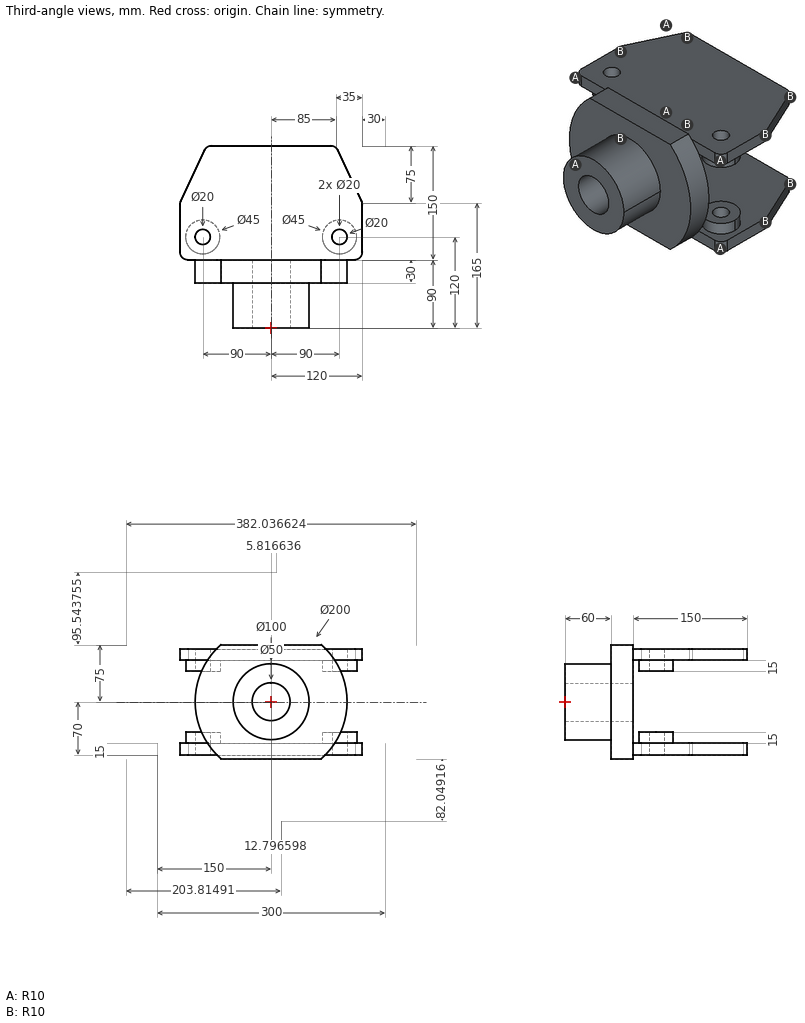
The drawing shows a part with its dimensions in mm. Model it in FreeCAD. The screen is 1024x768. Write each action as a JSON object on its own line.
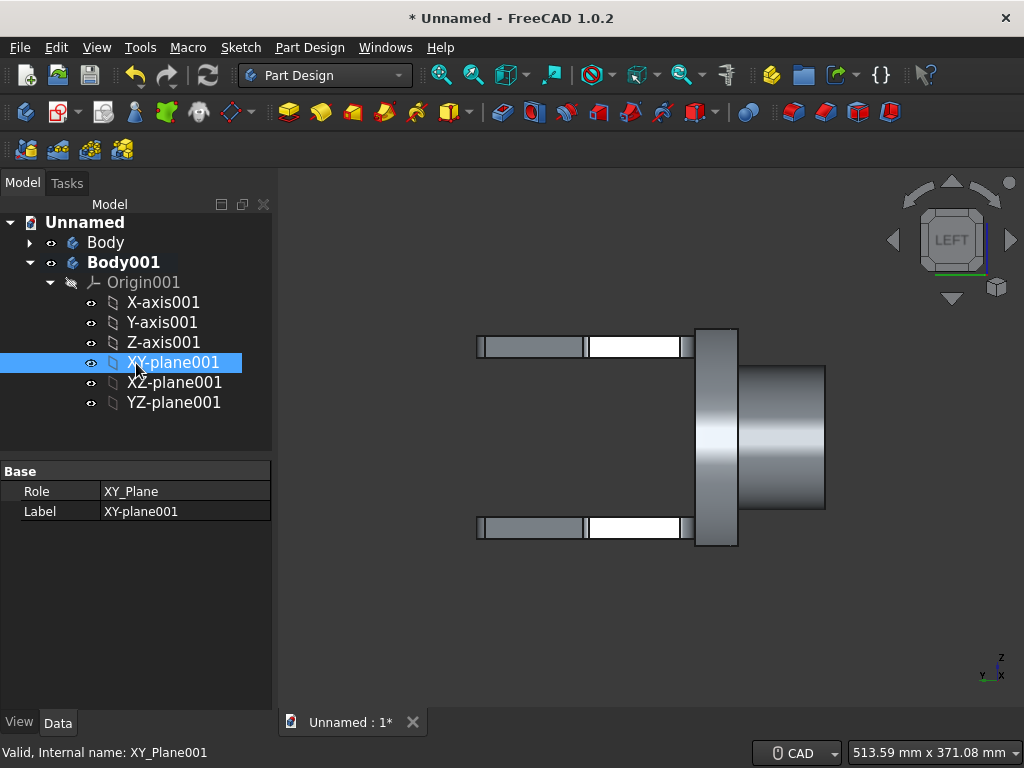
{"action": "left_click", "coordinate": [232, 112]}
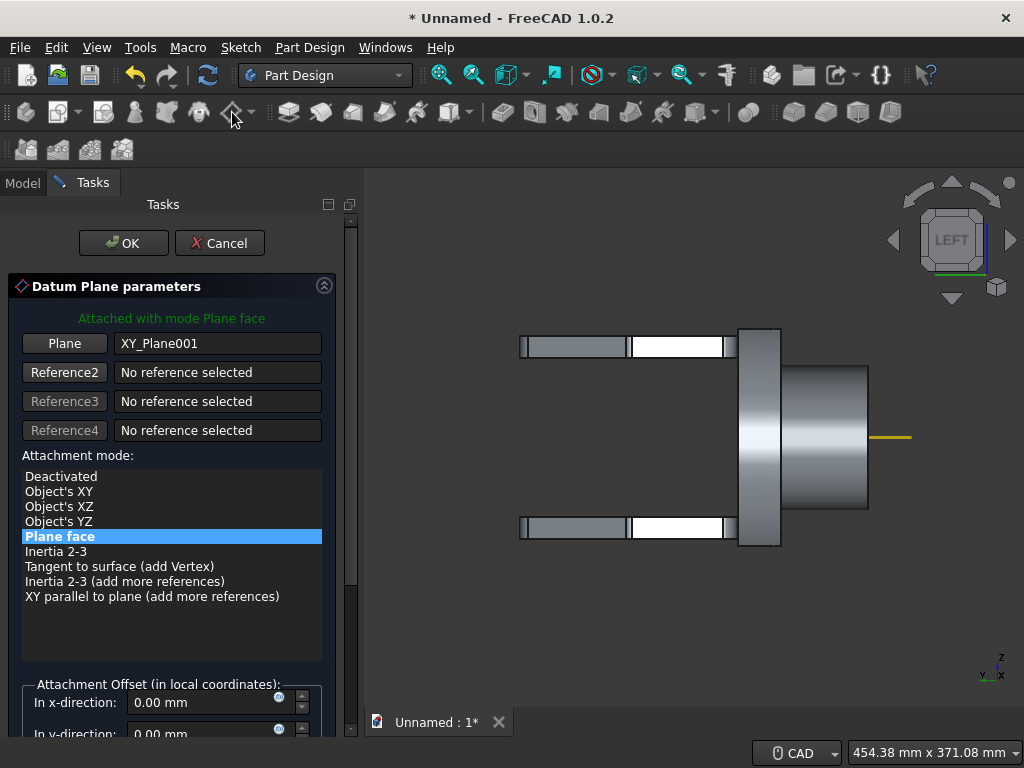
{"action": "scroll", "coordinate": [351, 475], "scroll_direction": "down", "scroll_amount": 2}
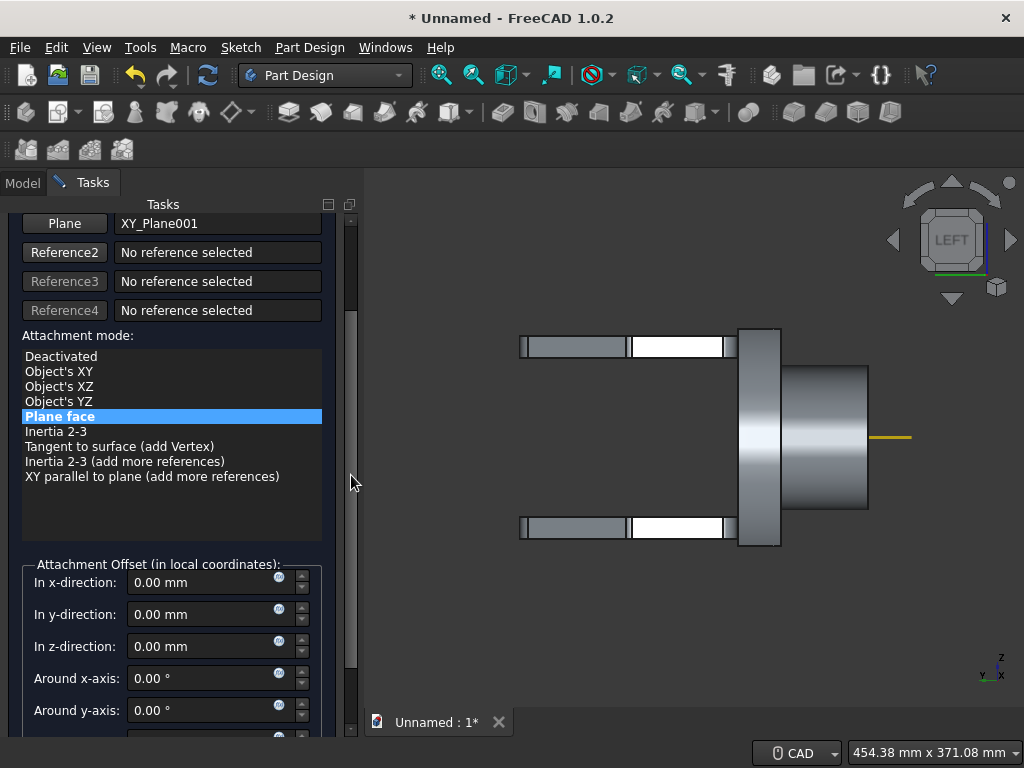
{"action": "triple_click", "coordinate": [210, 646]}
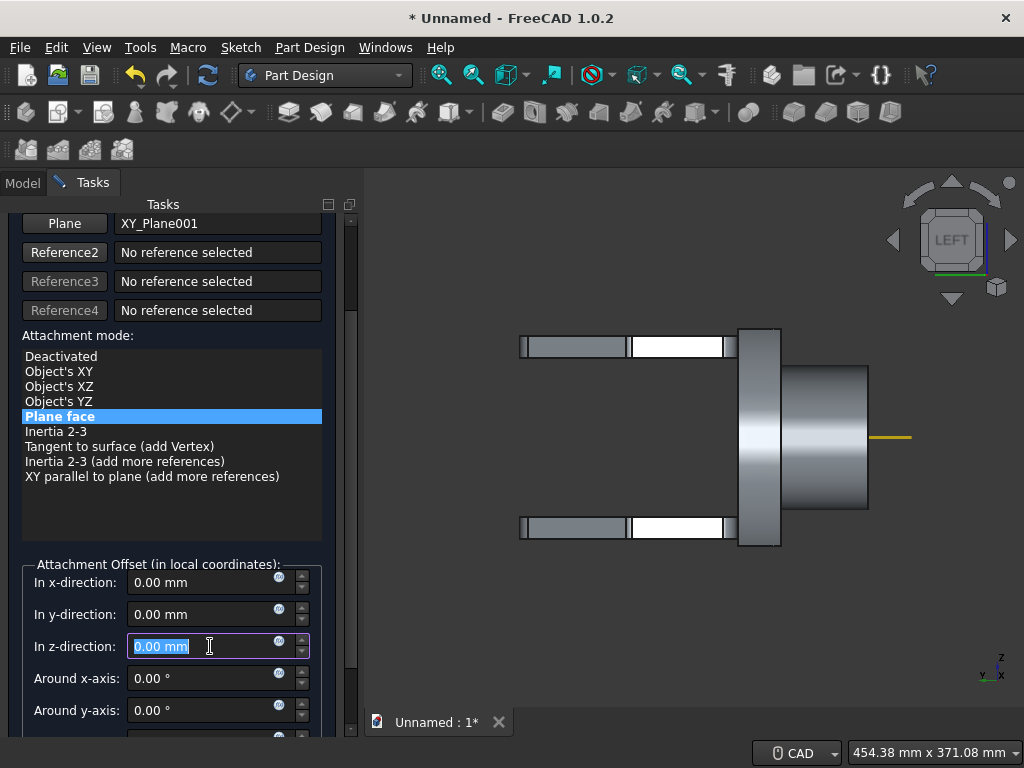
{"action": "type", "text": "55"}
{"action": "key", "text": "Tab"}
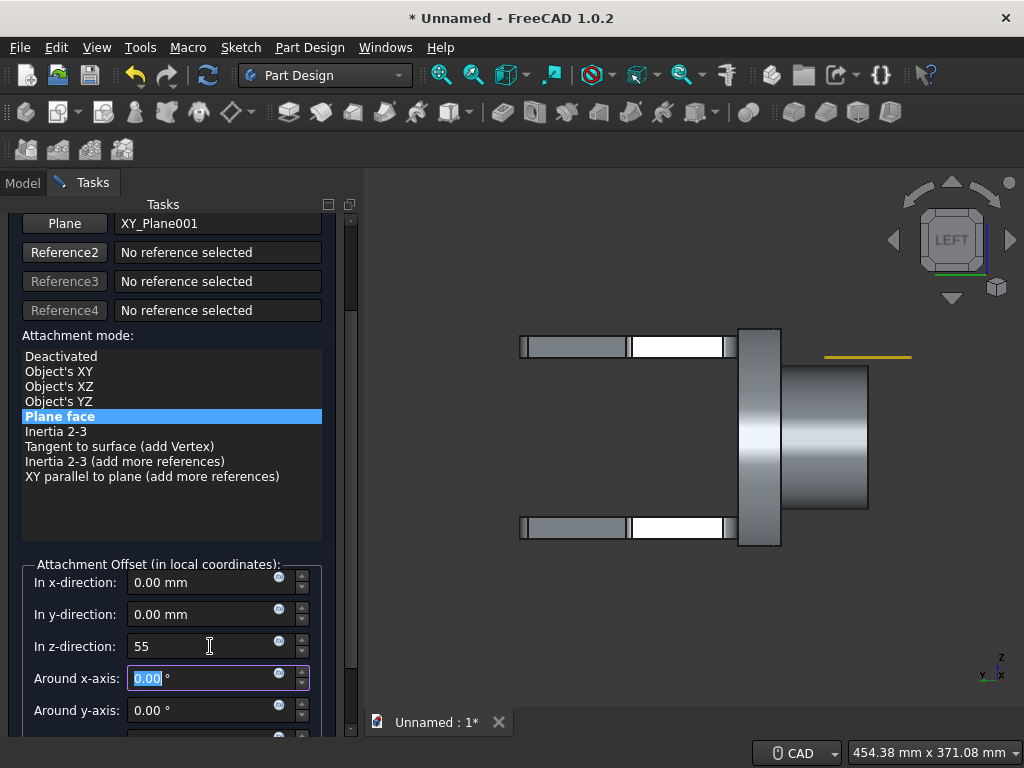
{"action": "scroll", "coordinate": [351, 475], "scroll_direction": "up", "scroll_amount": 3}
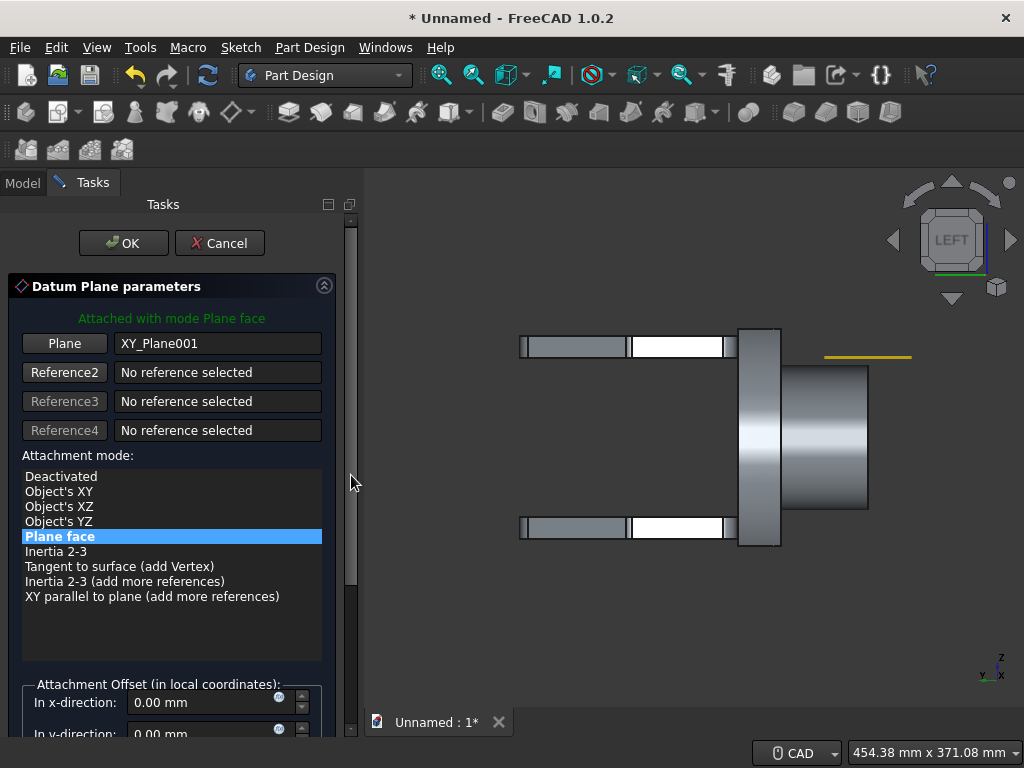
{"action": "left_click", "coordinate": [124, 243]}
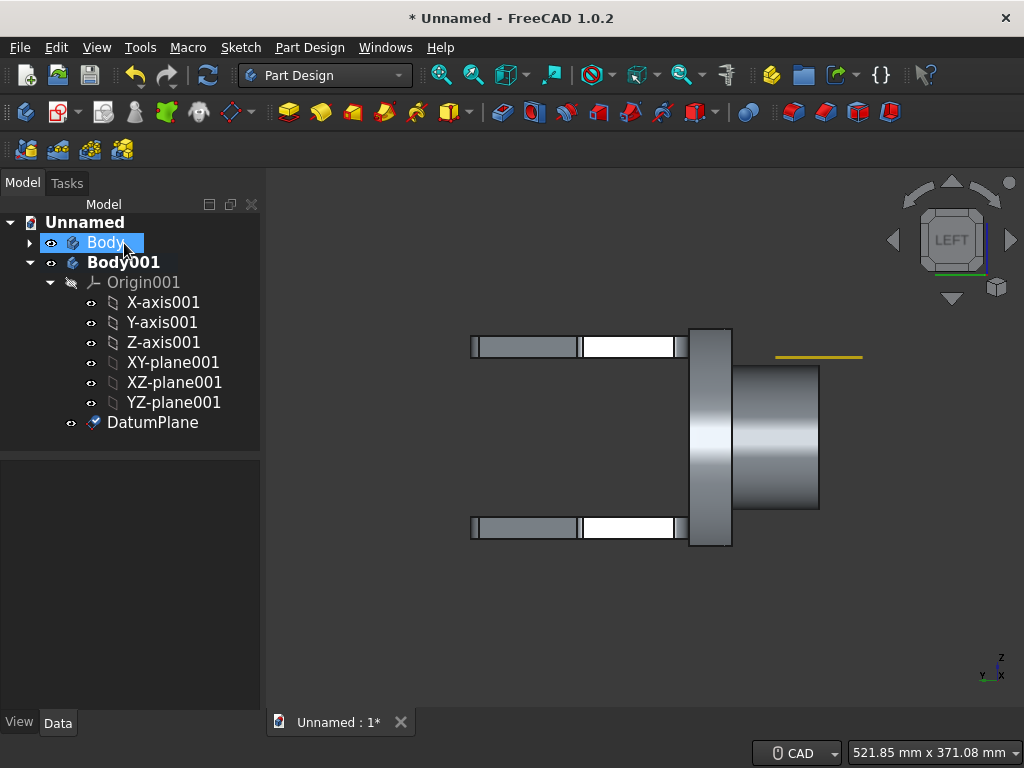
{"action": "left_click", "coordinate": [116, 423]}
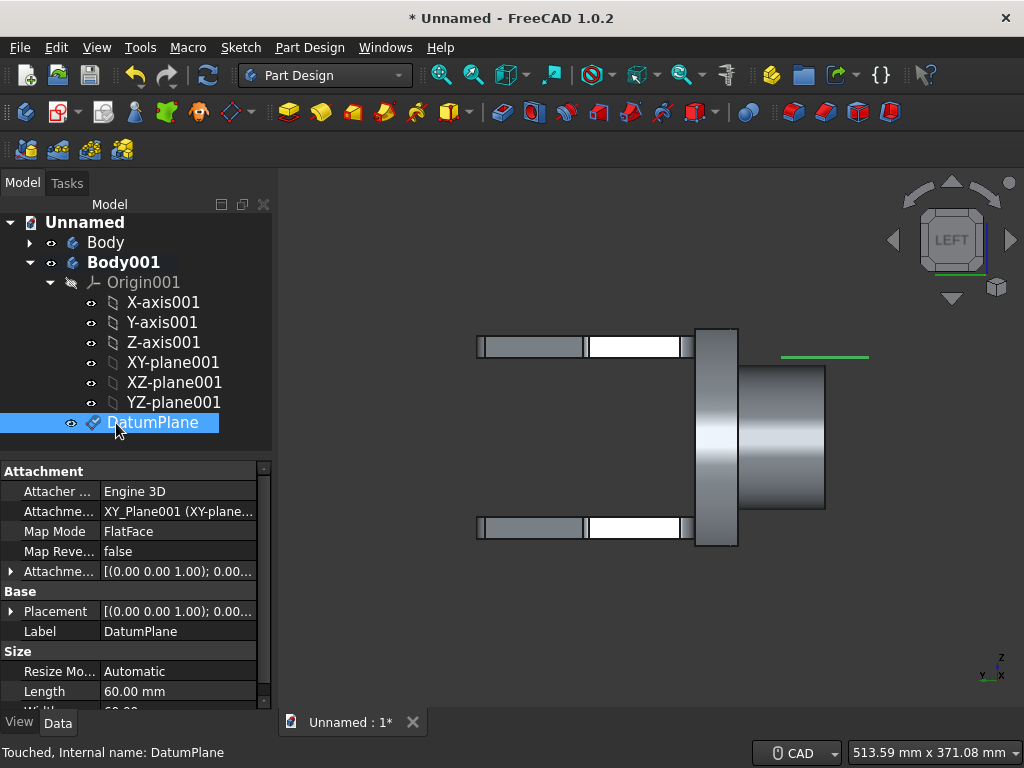
{"action": "left_click", "coordinate": [58, 112]}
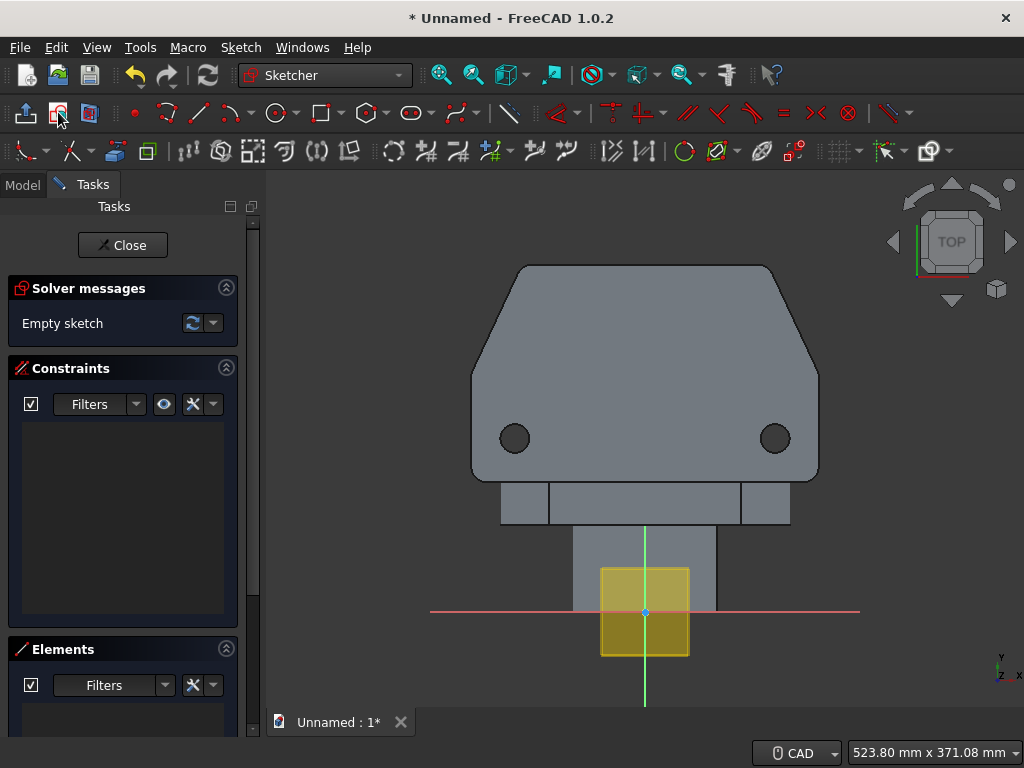
{"action": "scroll", "coordinate": [499, 439], "scroll_direction": "up", "scroll_amount": 8}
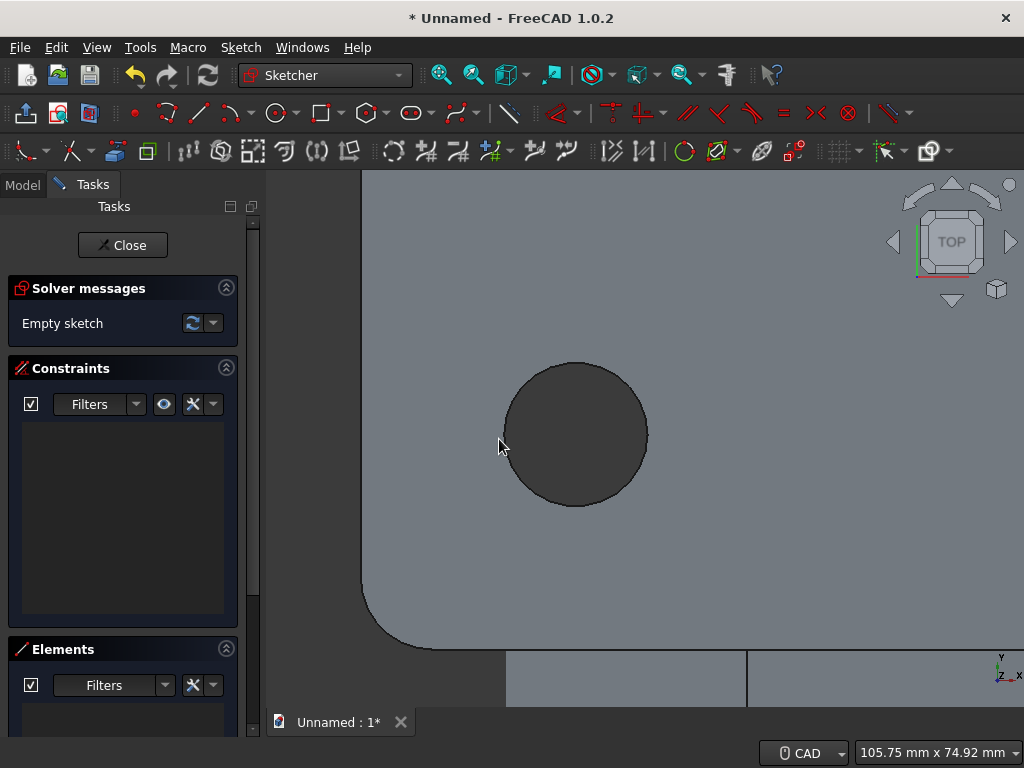
{"action": "key", "text": "g c"}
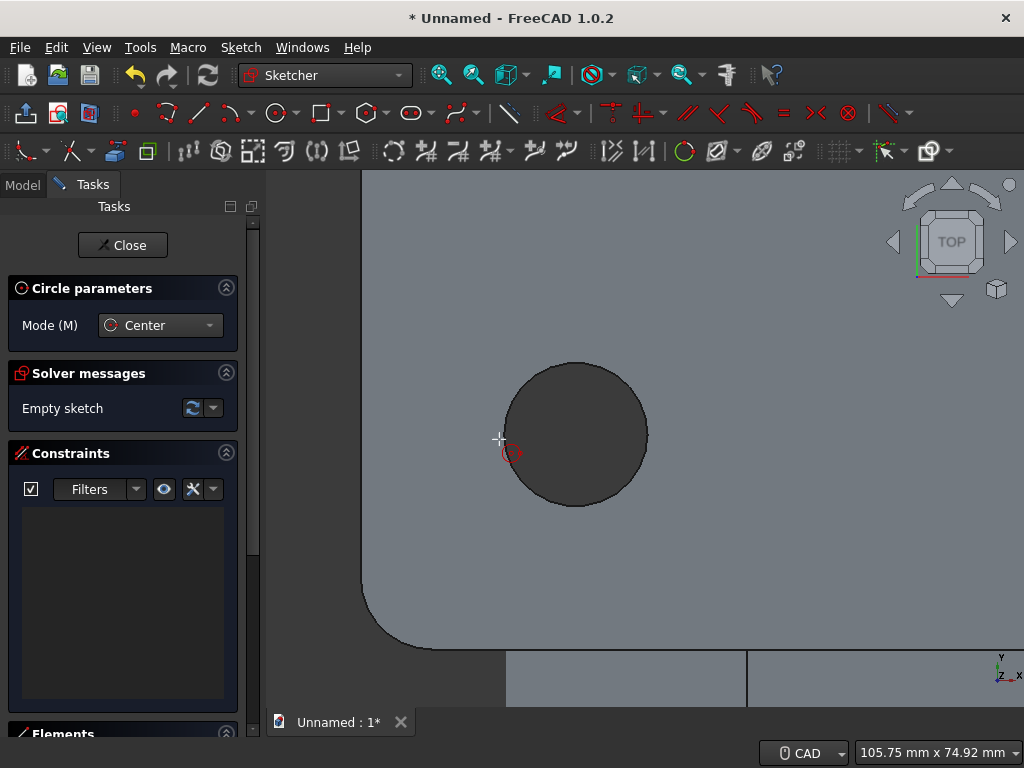
{"action": "left_click", "coordinate": [576, 435]}
{"action": "left_click", "coordinate": [690, 321]}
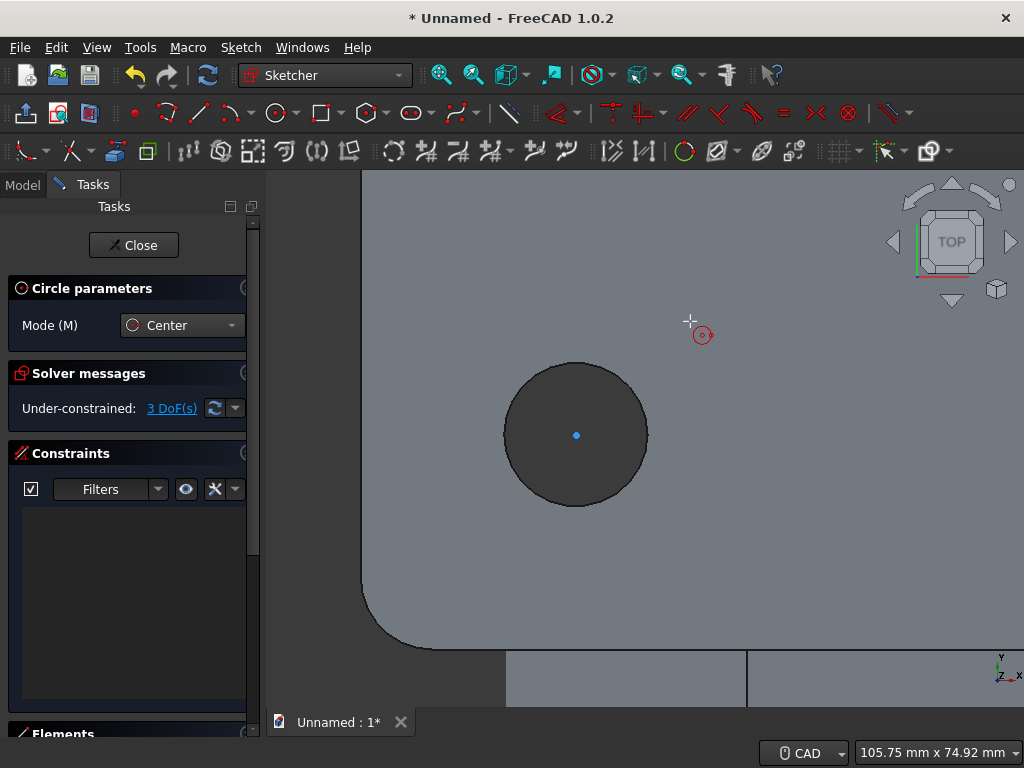
{"action": "left_click", "coordinate": [576, 436]}
{"action": "left_click", "coordinate": [627, 384]}
{"action": "key", "text": "Escape"}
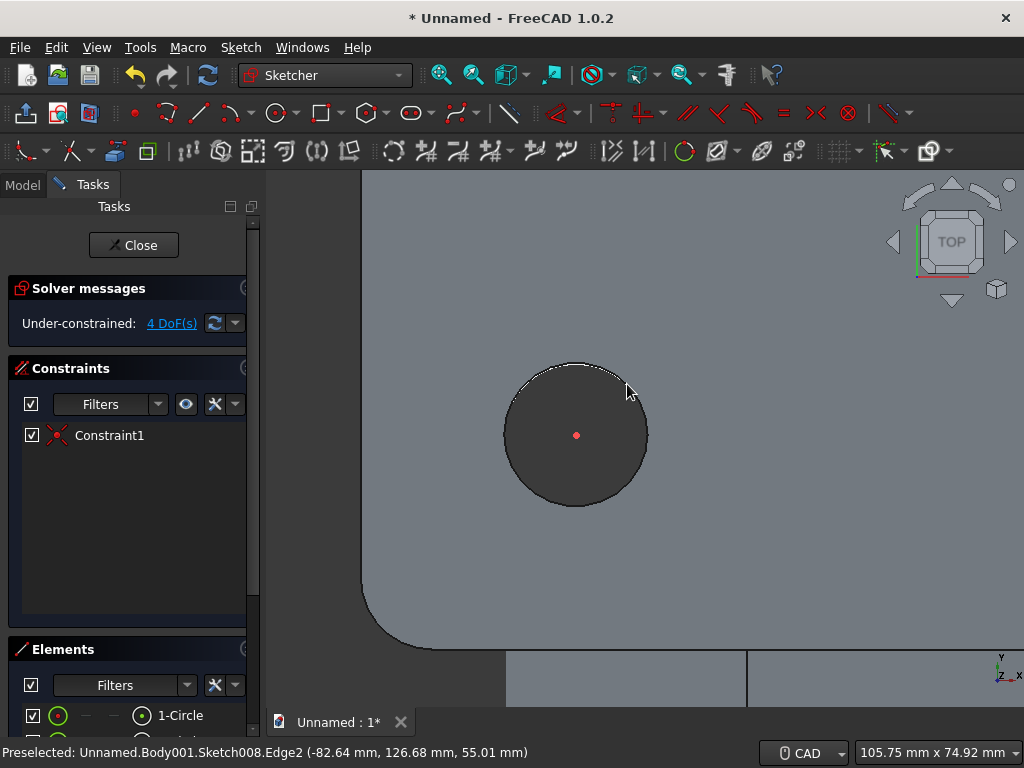
{"action": "left_click", "coordinate": [556, 114]}